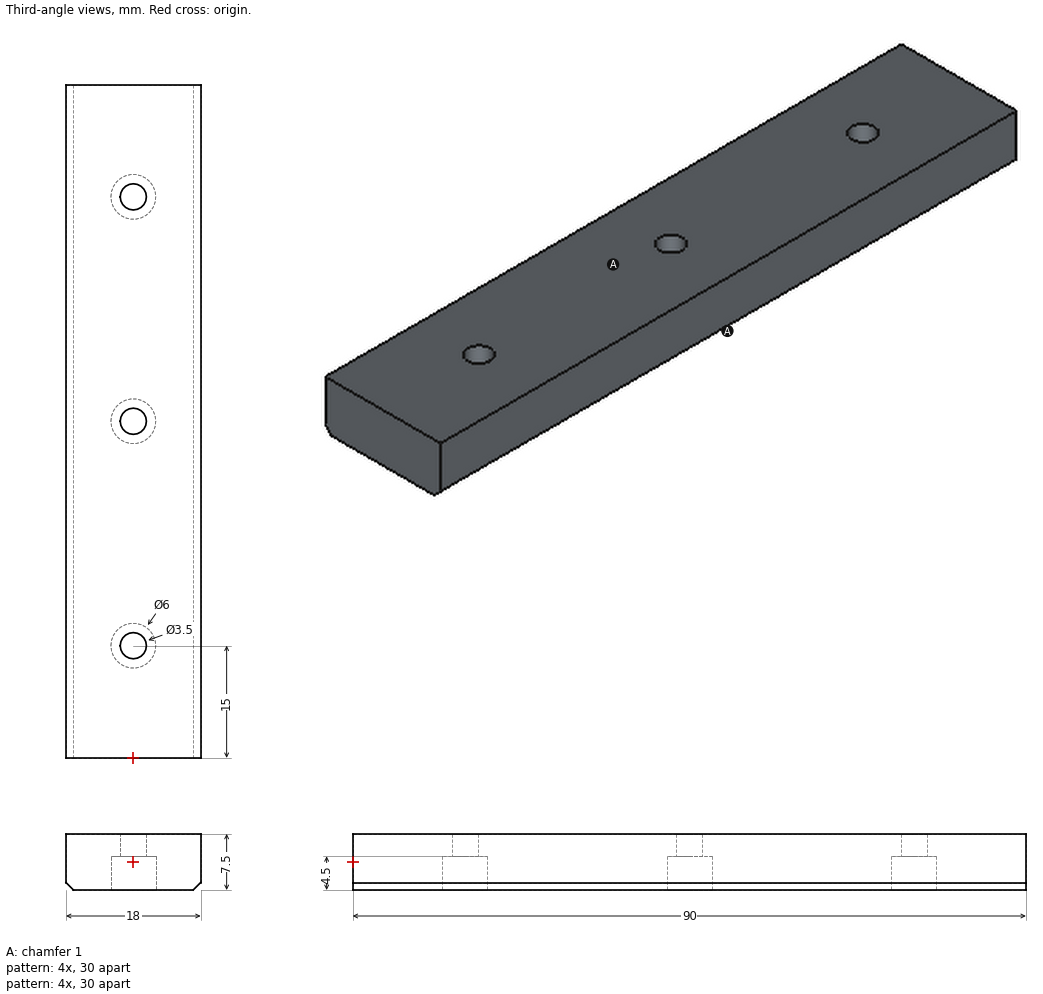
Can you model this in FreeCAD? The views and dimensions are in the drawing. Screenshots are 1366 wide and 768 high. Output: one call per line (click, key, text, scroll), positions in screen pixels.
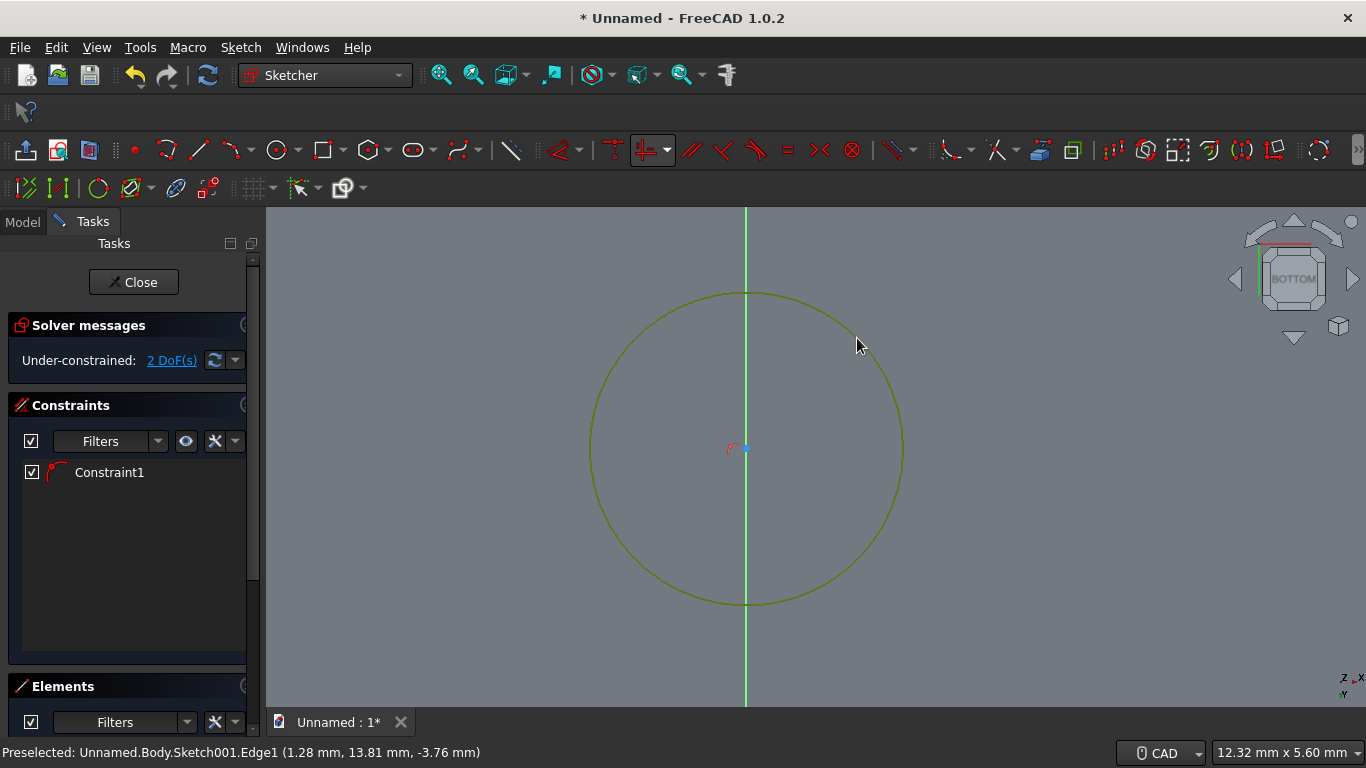
click(582, 150)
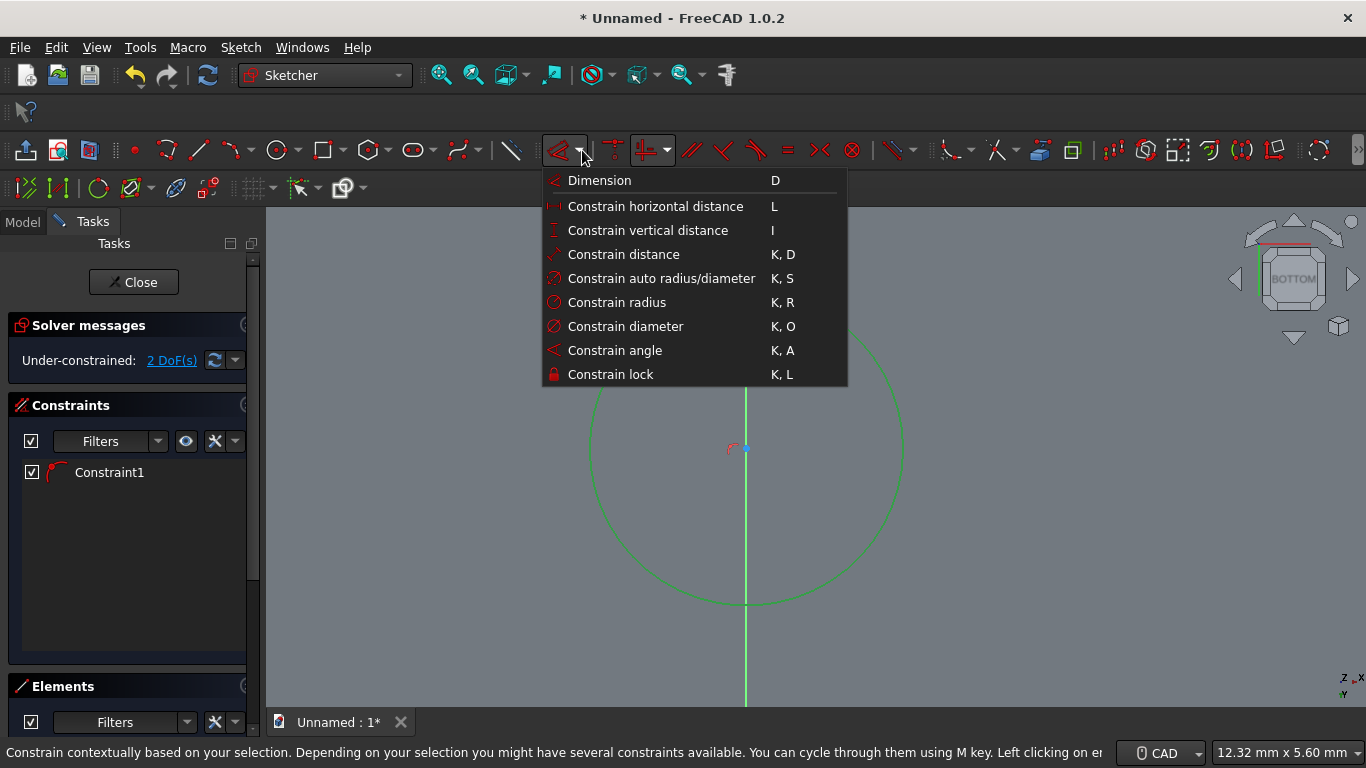
click(695, 326)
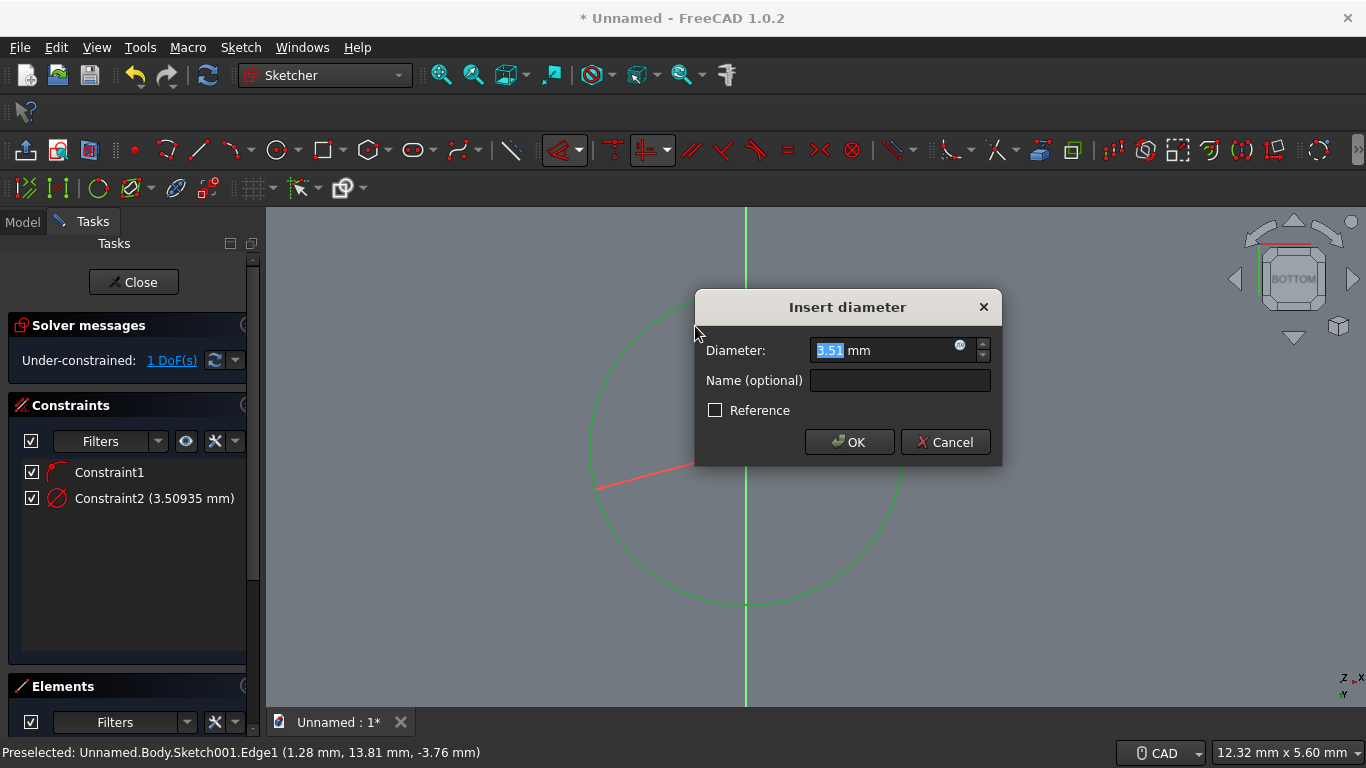
text(3.5)
key(Return)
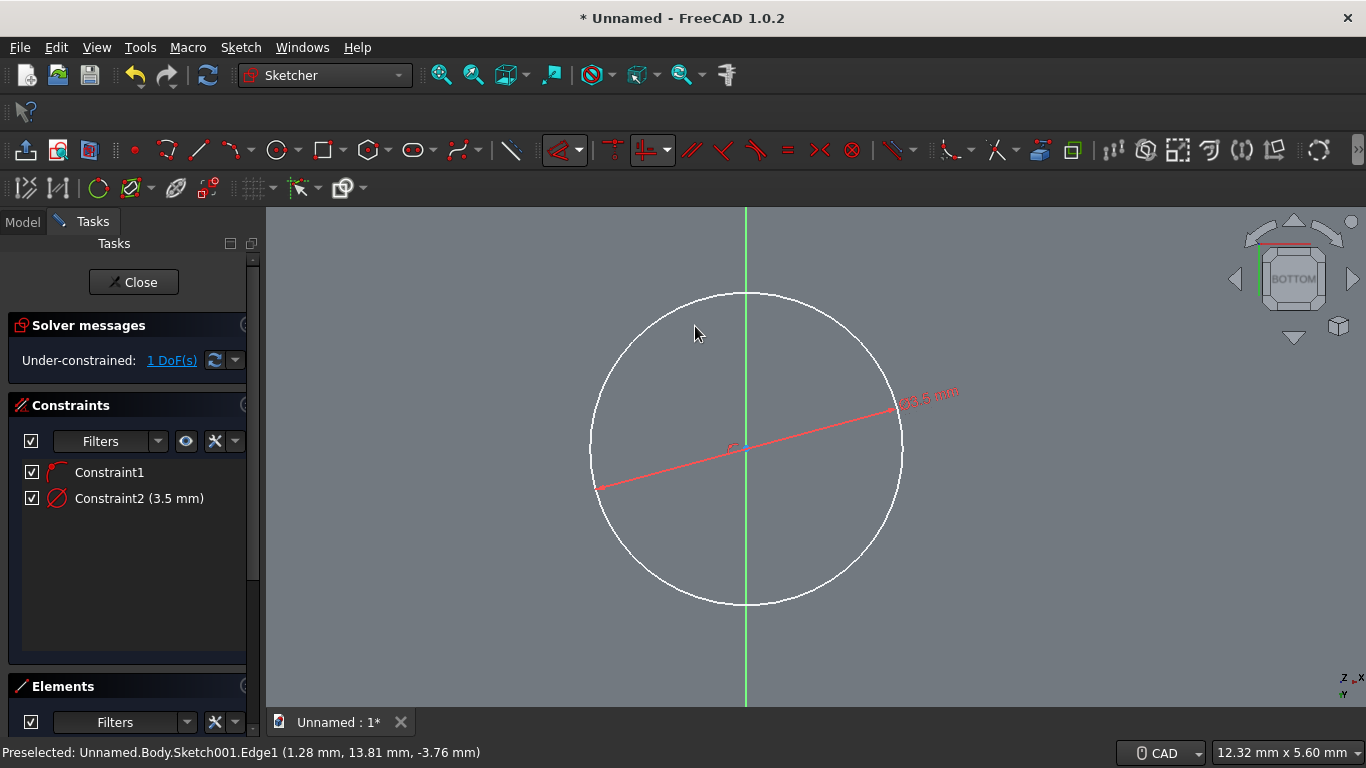
click(746, 449)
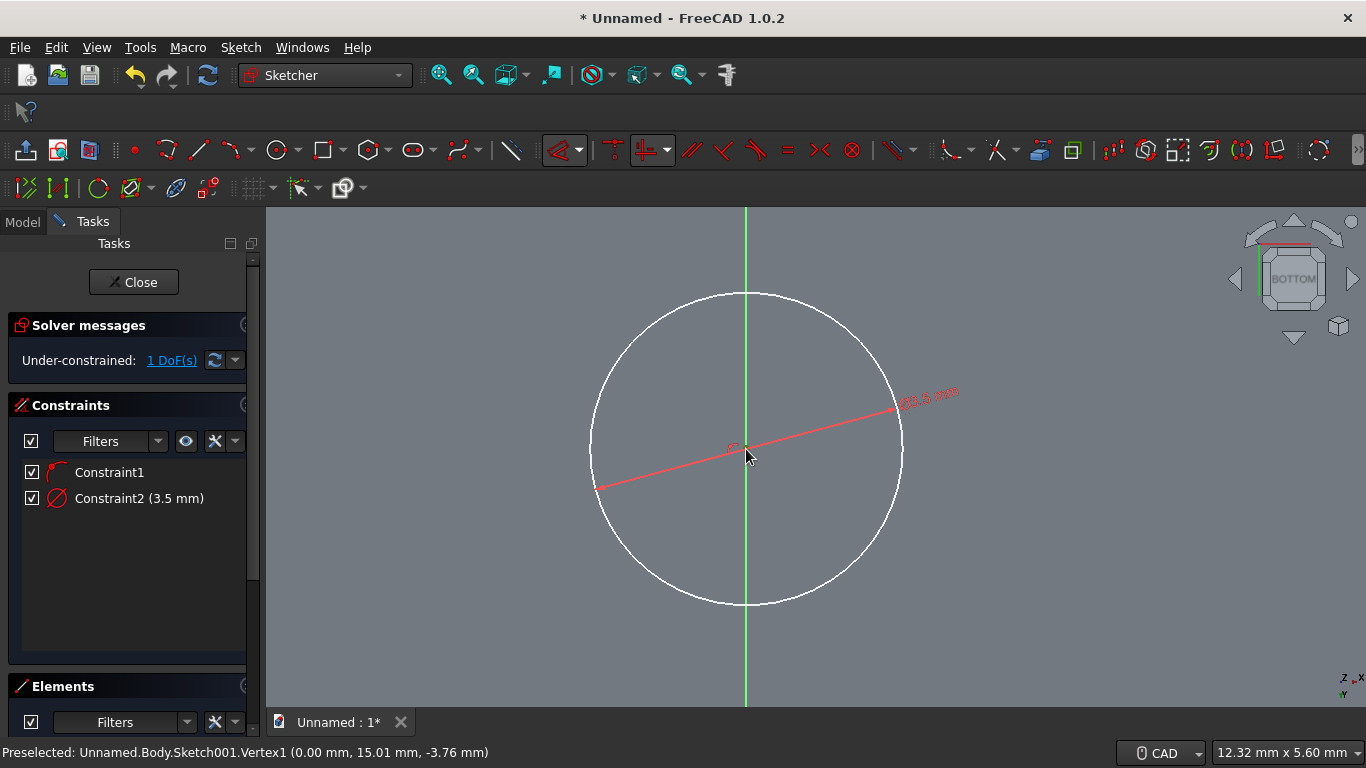
click(582, 150)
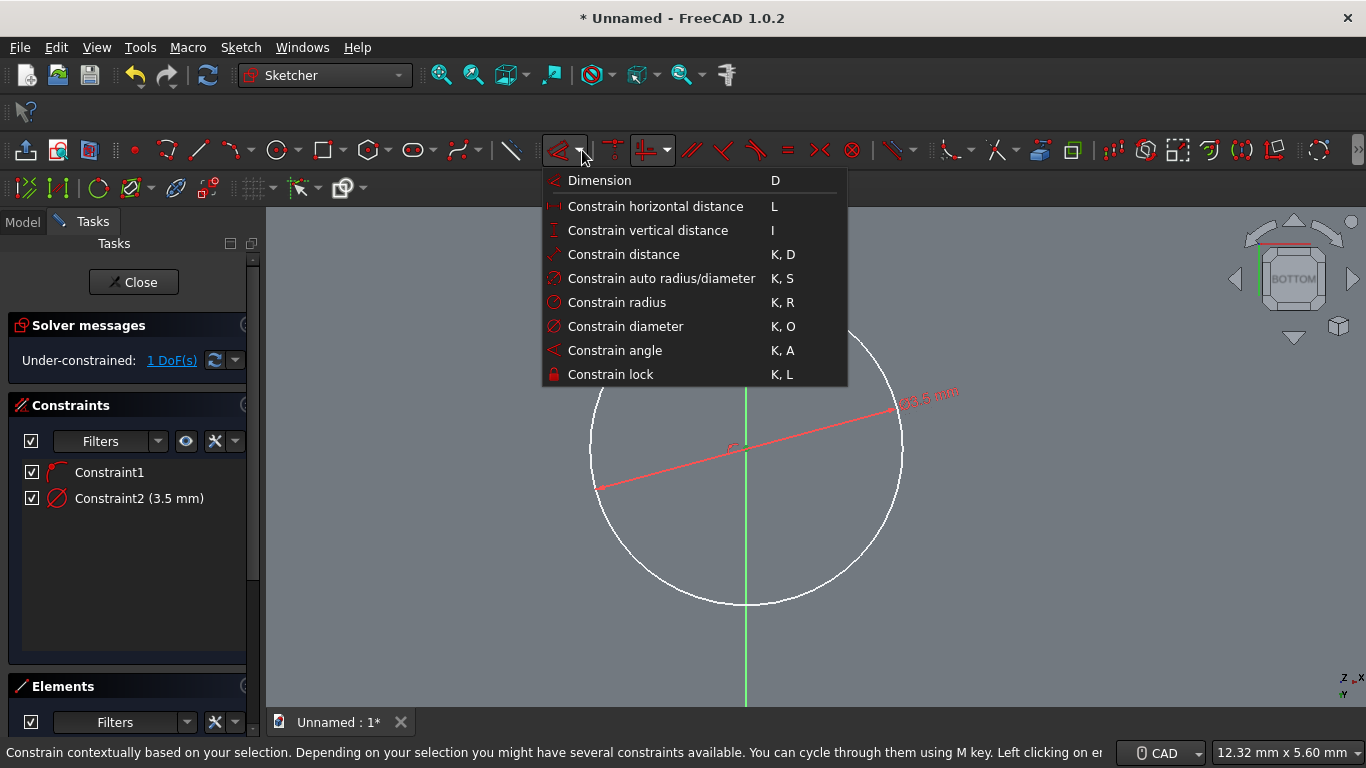
click(695, 230)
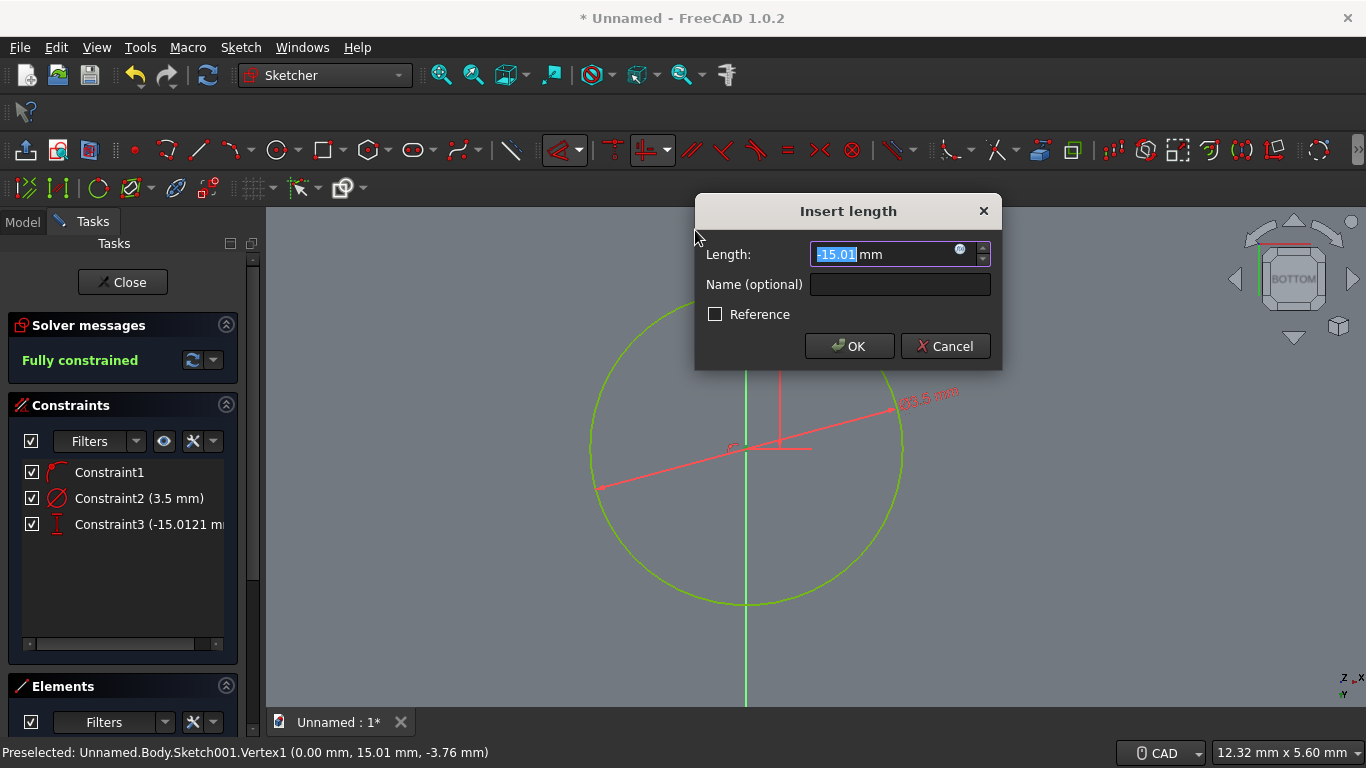
text(-15)
key(Return)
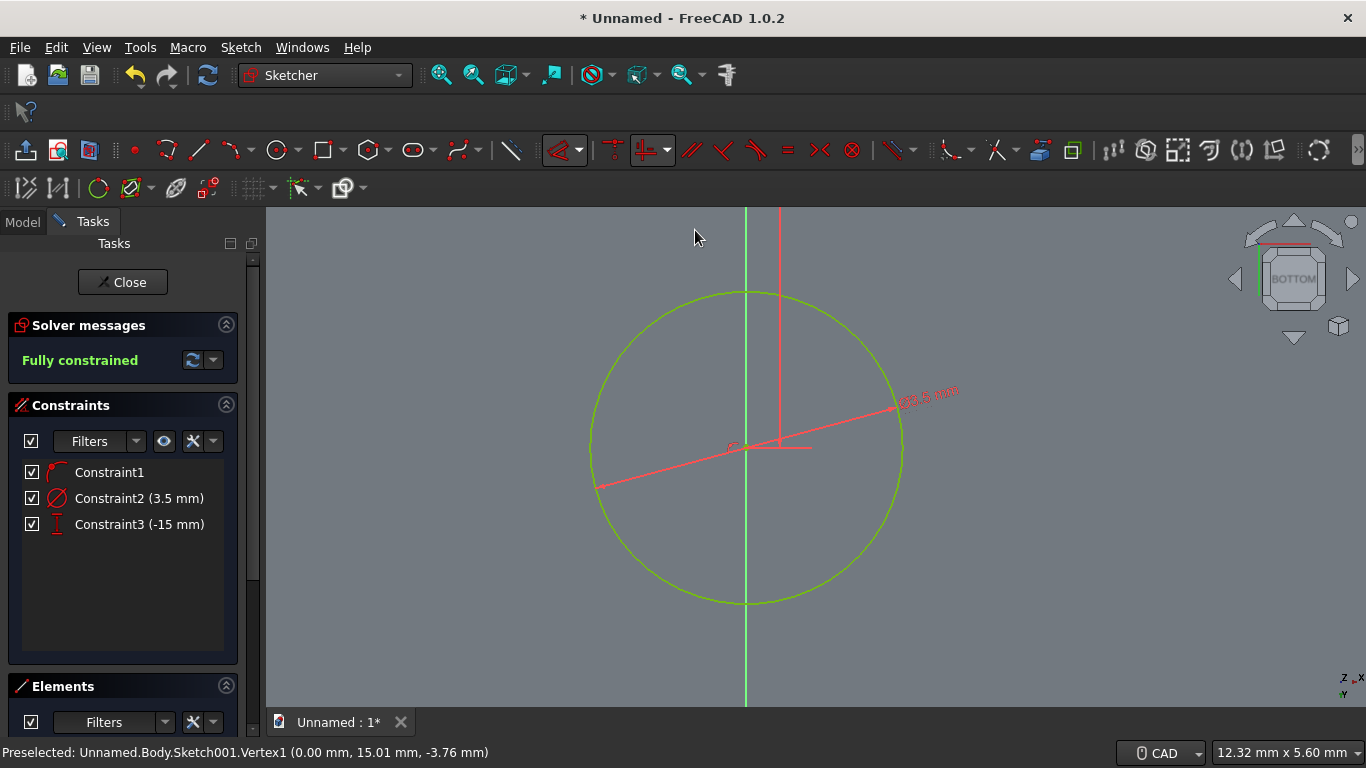
click(123, 282)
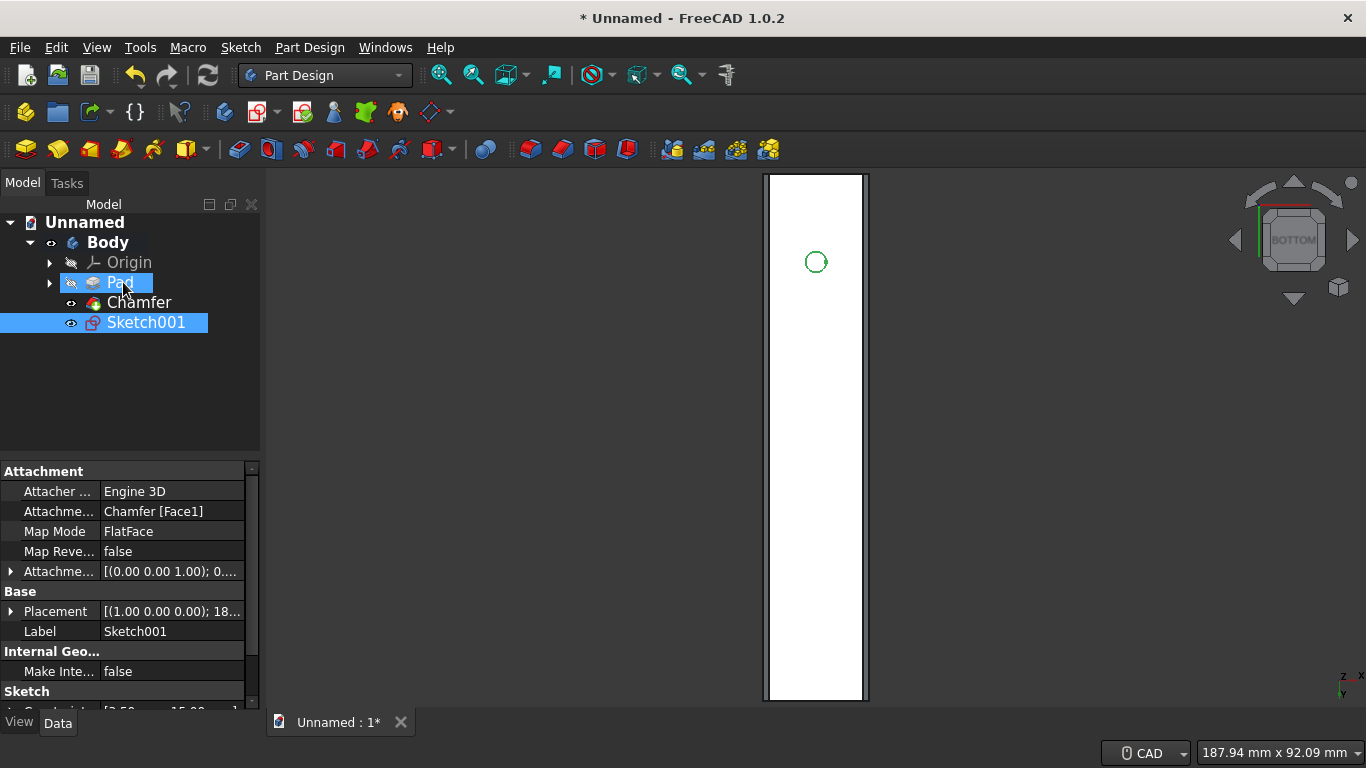
click(240, 150)